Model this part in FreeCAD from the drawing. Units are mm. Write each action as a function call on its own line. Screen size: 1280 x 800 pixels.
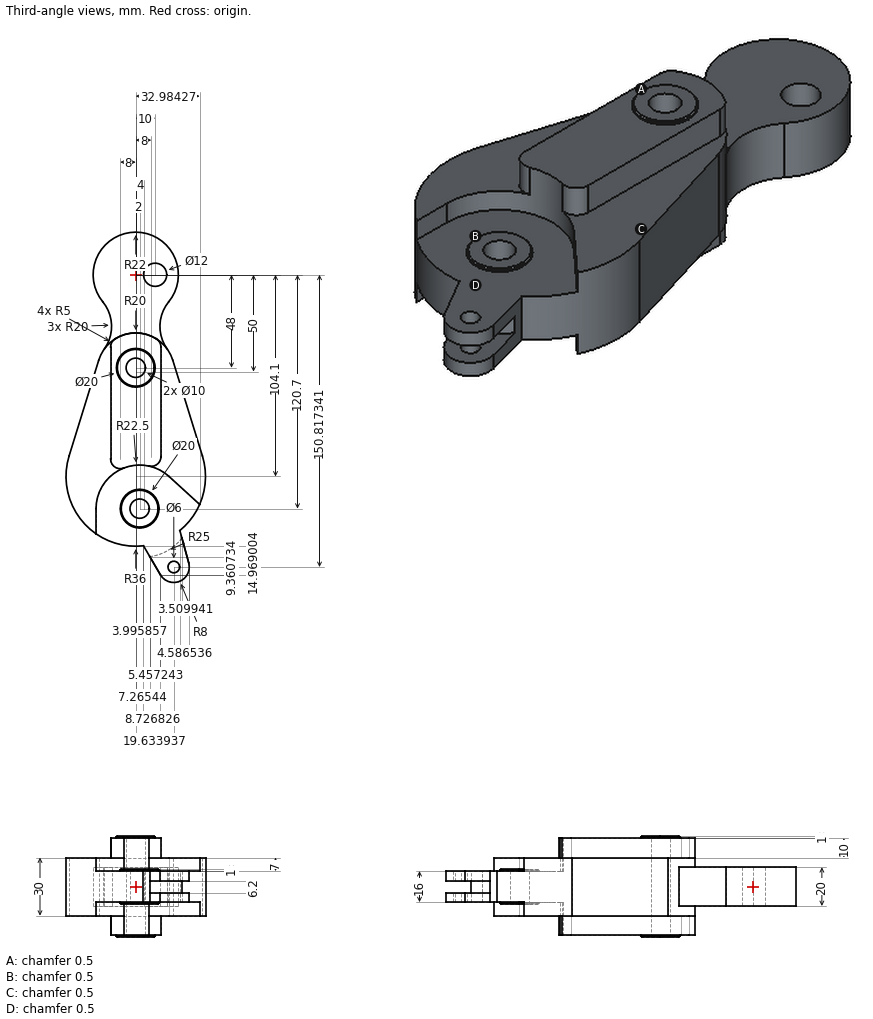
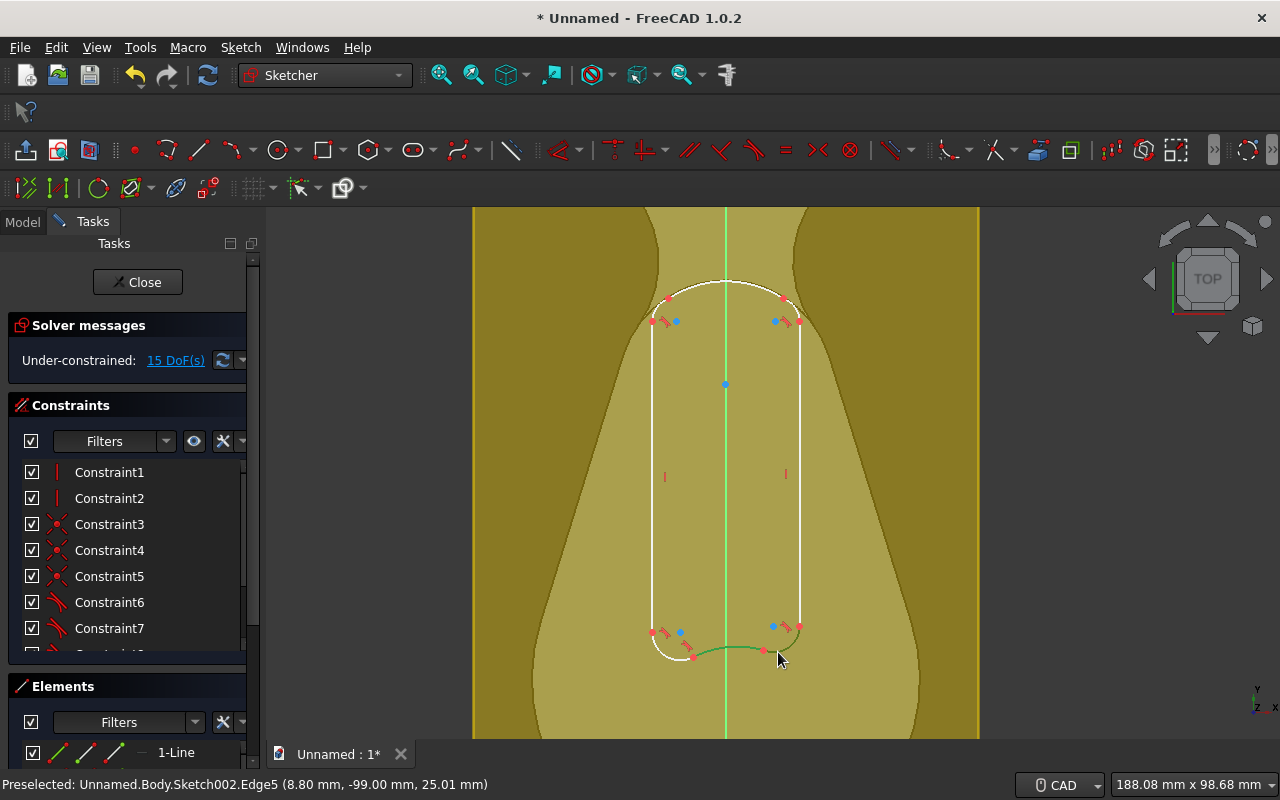
click(754, 150)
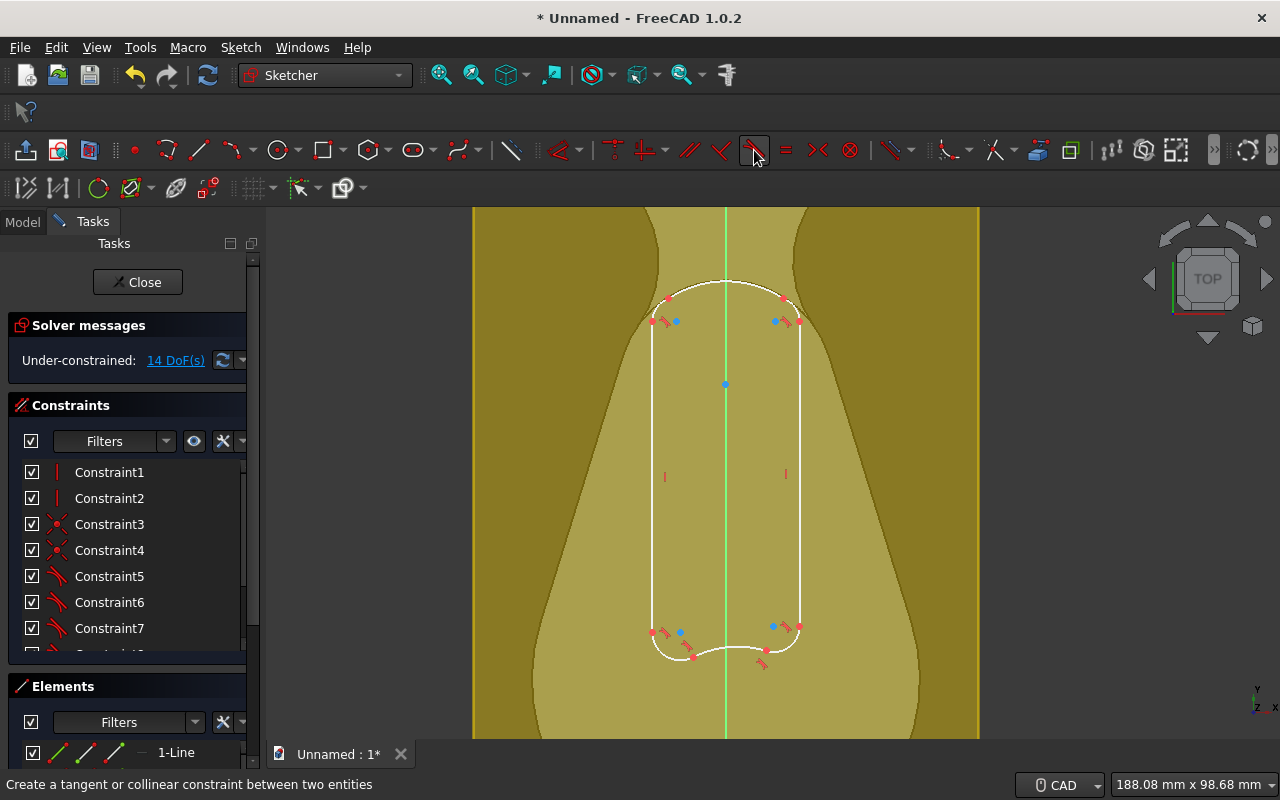
click(795, 308)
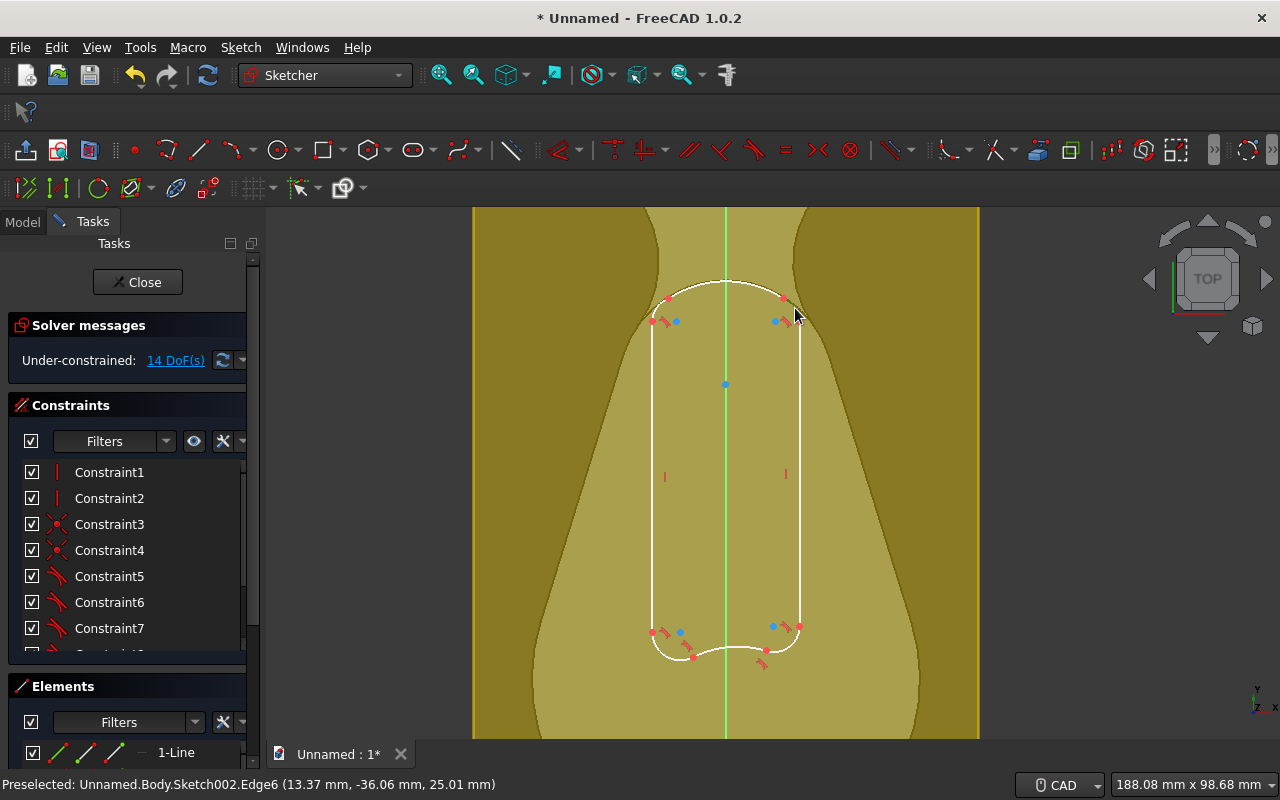
click(750, 284)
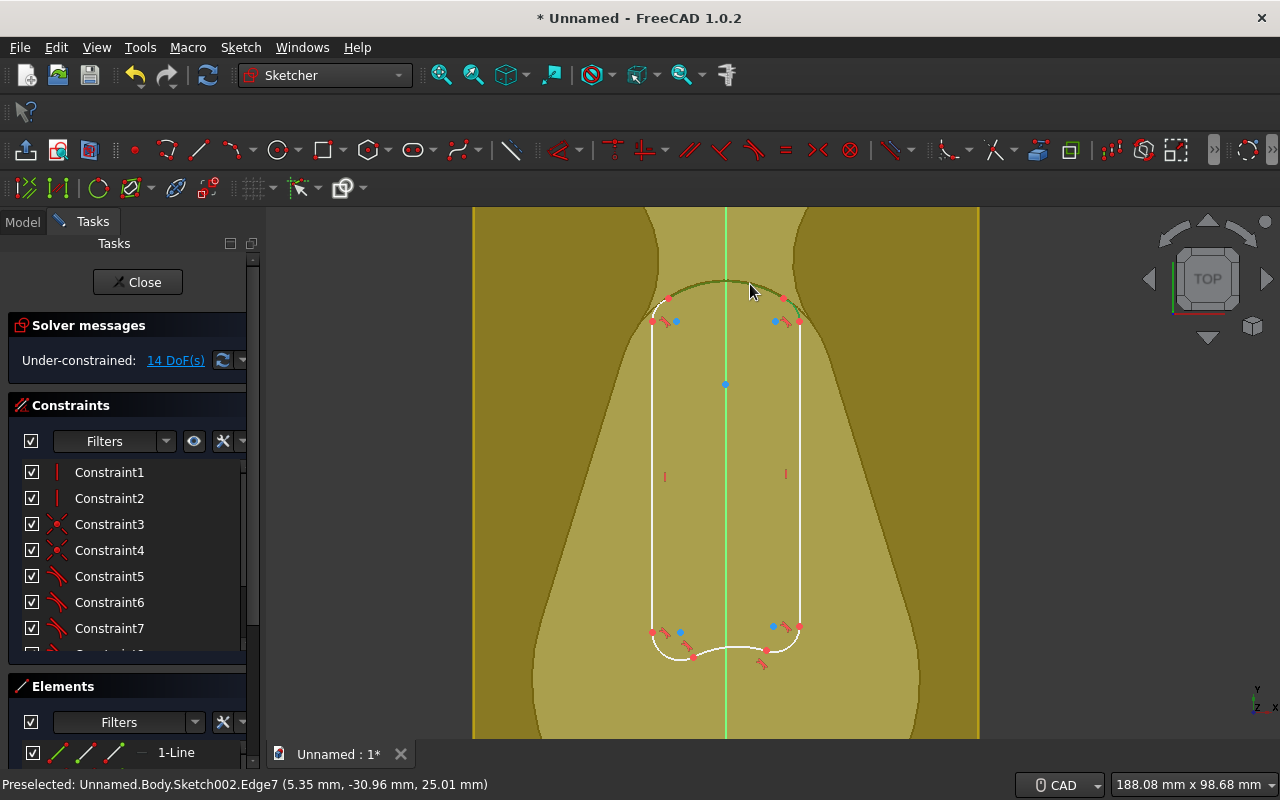
click(754, 150)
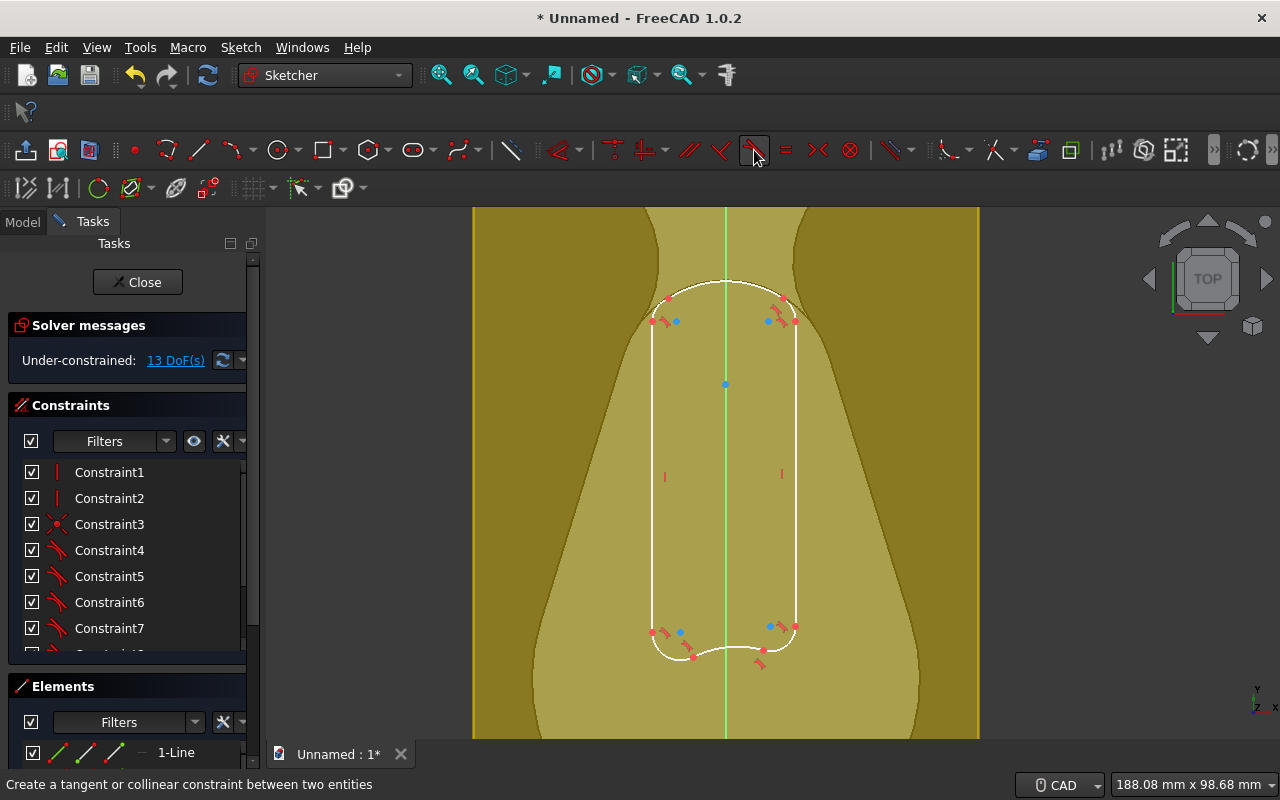
click(750, 284)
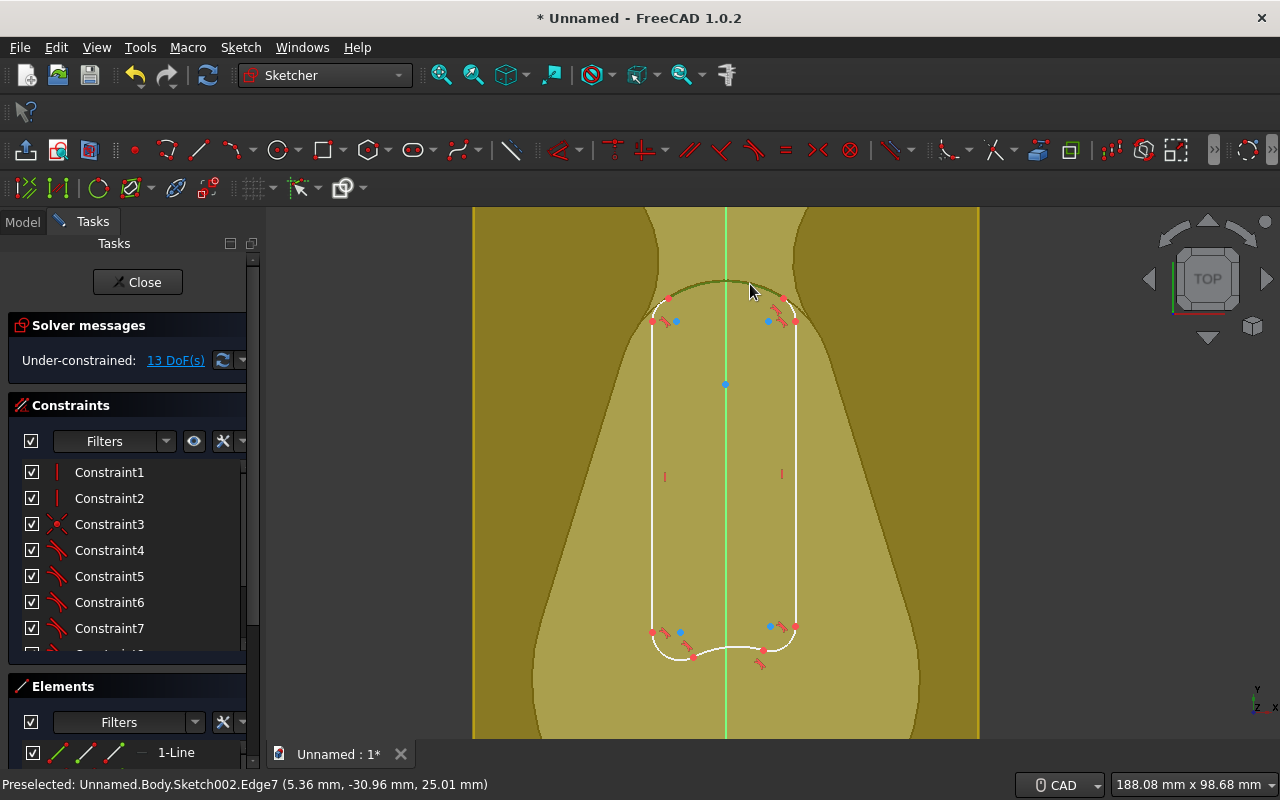
click(657, 308)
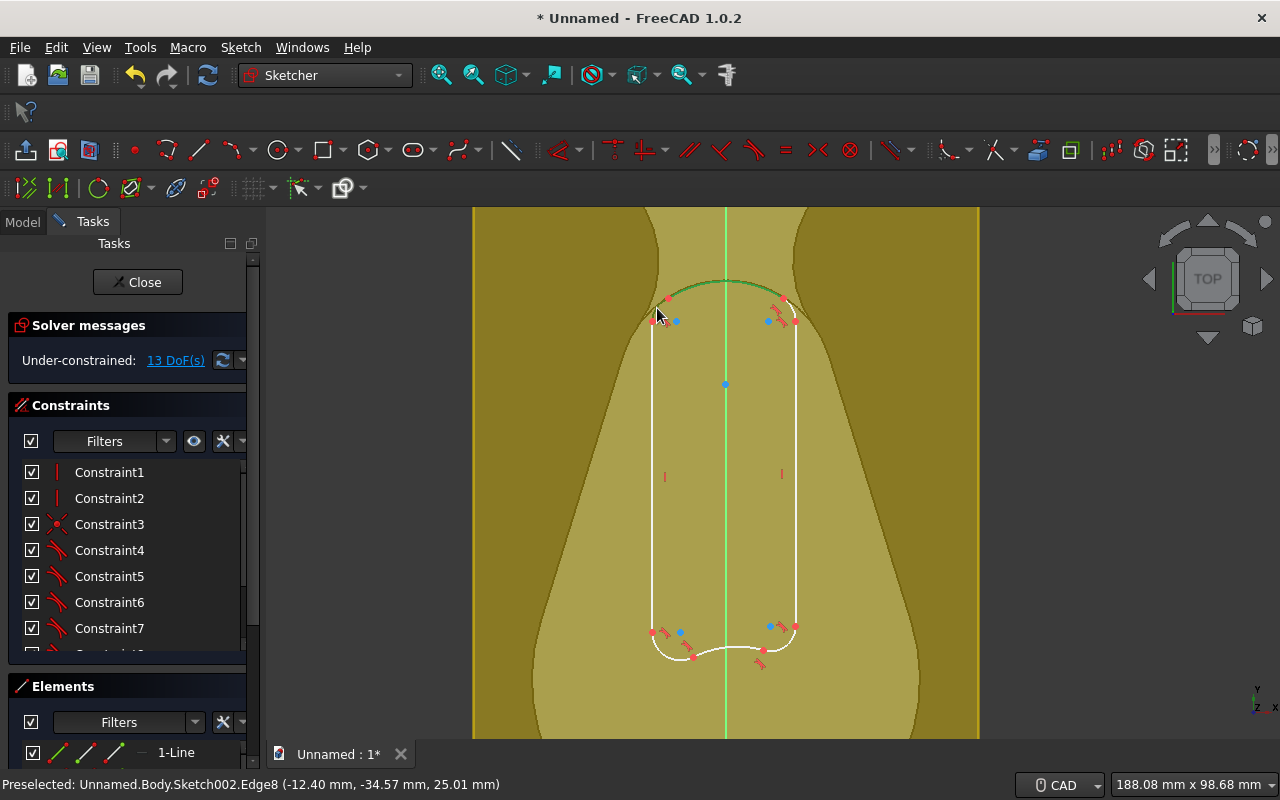
click(754, 150)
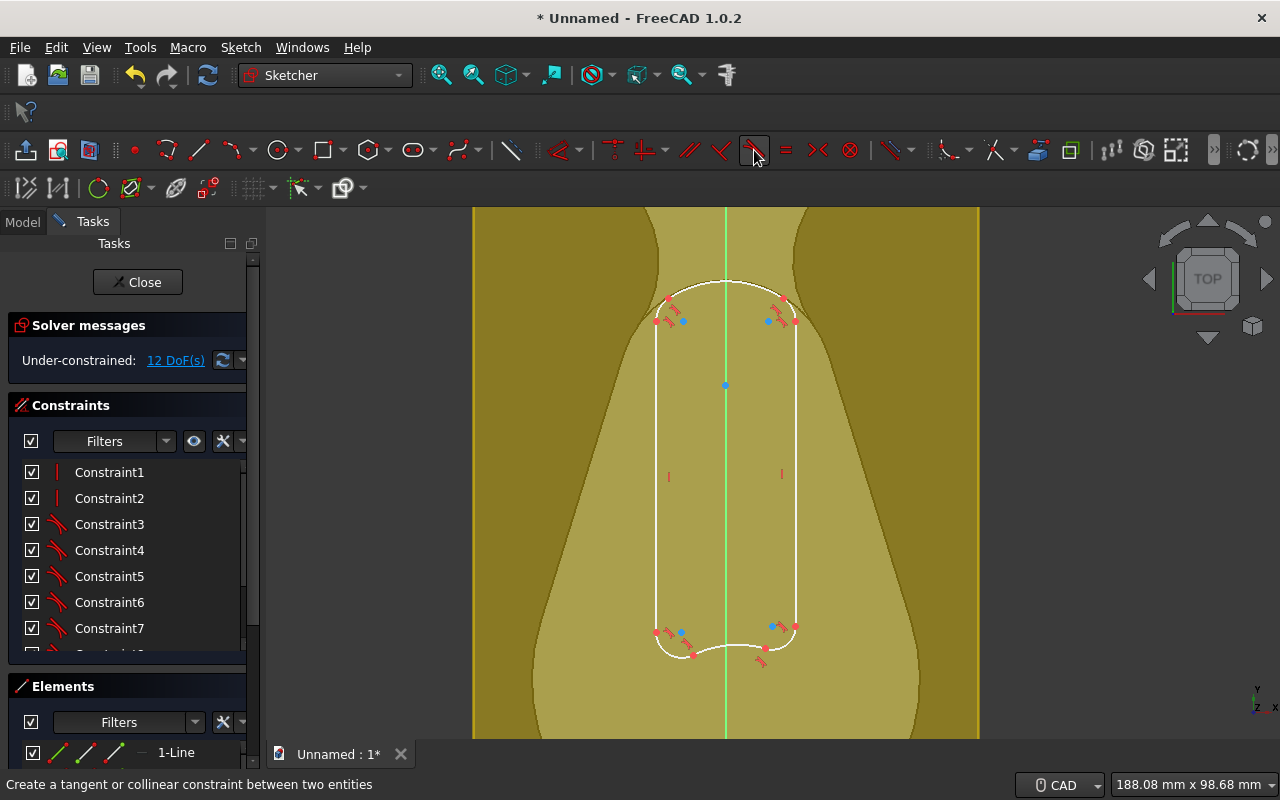
click(661, 647)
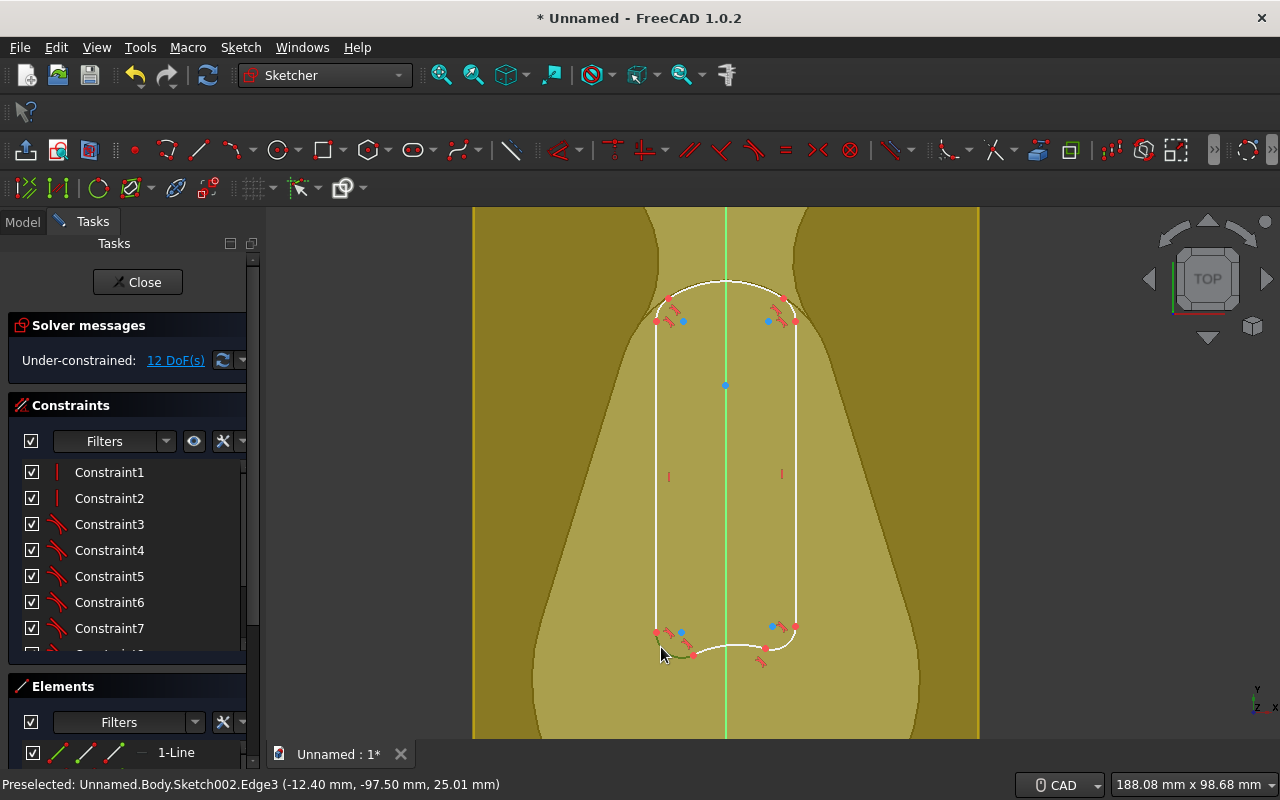
click(779, 649)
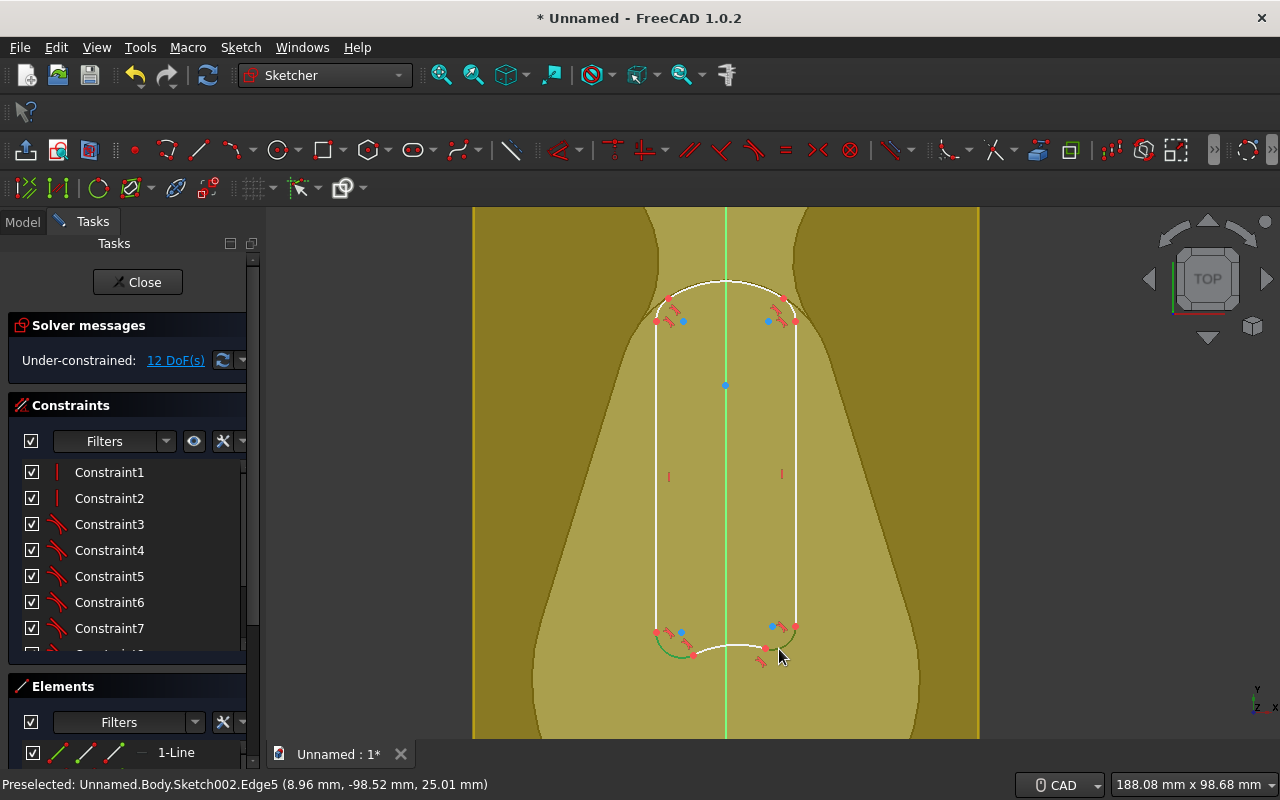
click(792, 309)